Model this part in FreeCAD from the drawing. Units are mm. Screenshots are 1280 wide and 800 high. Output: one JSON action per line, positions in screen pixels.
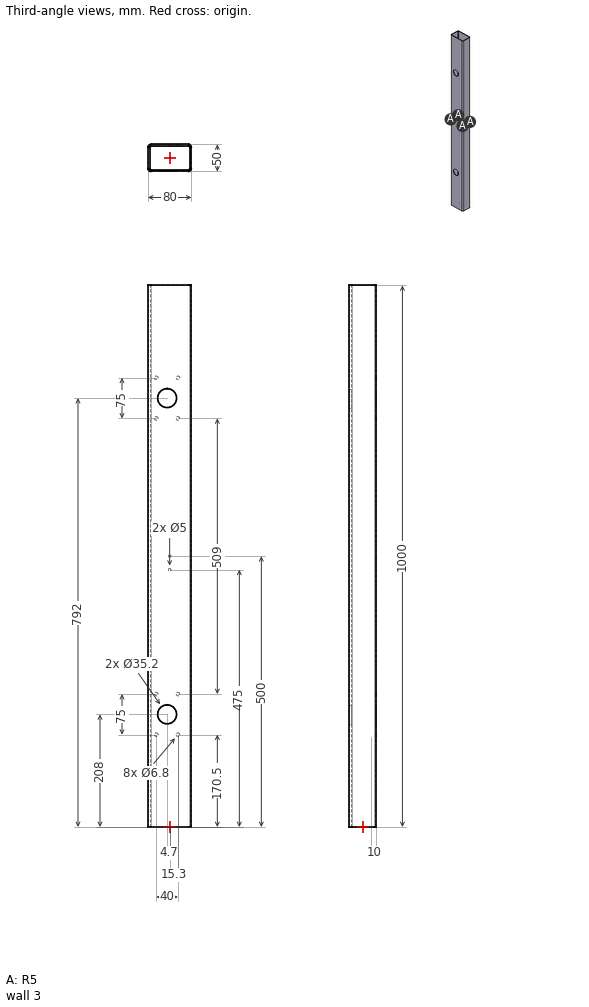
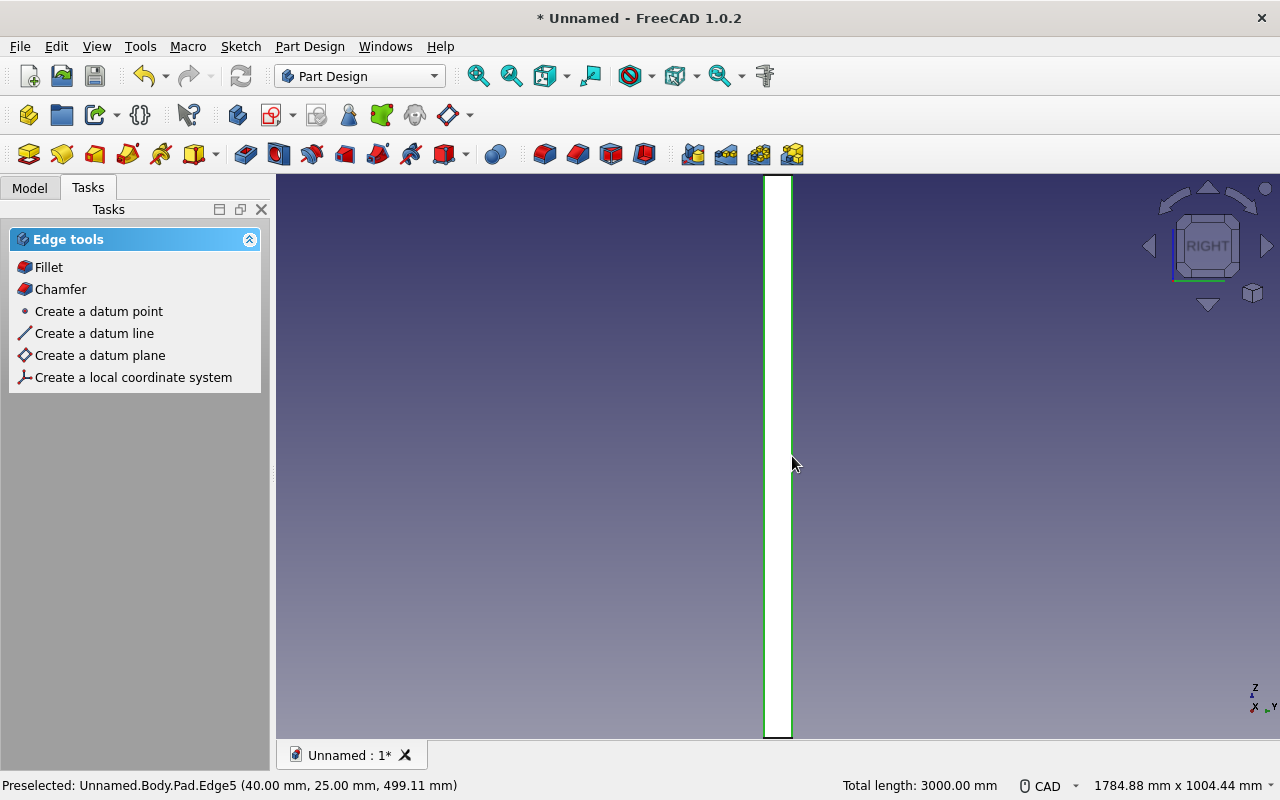
{"action": "key", "text": "5"}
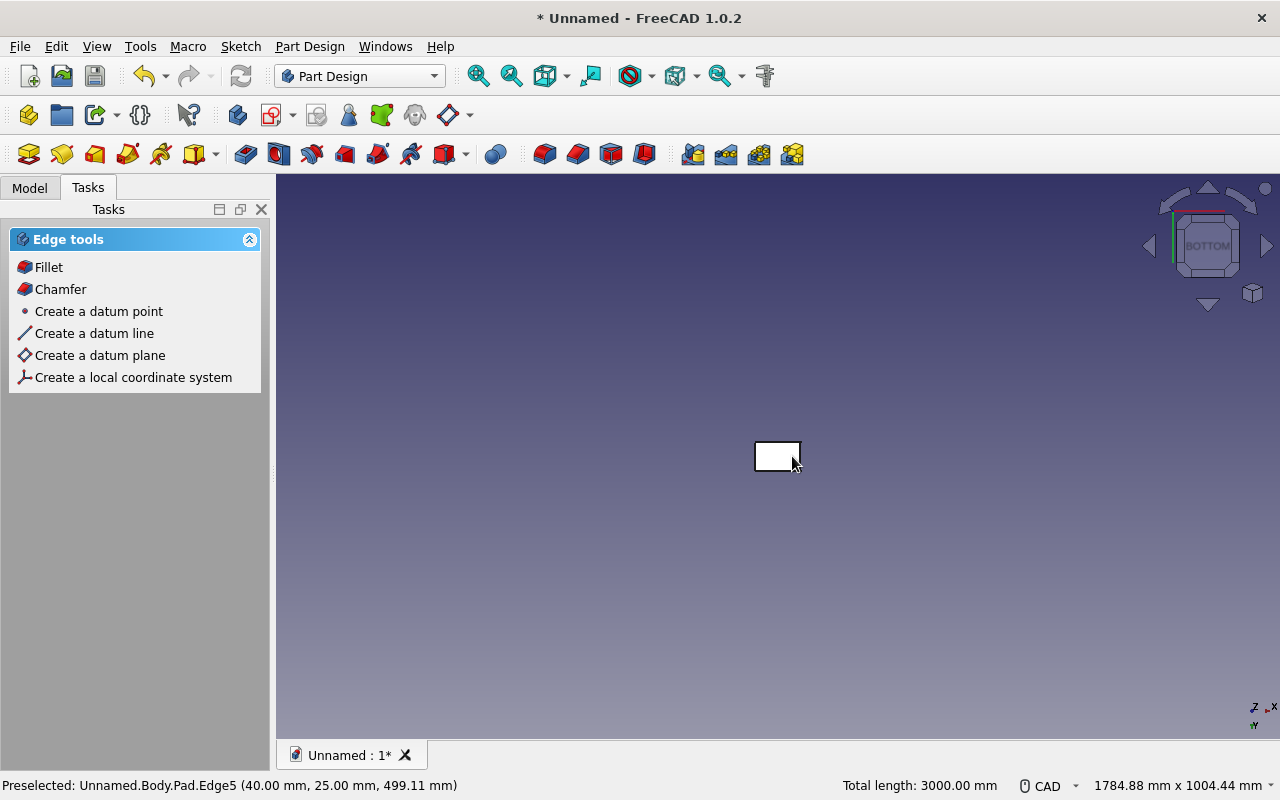
{"action": "left_click", "coordinate": [479, 76]}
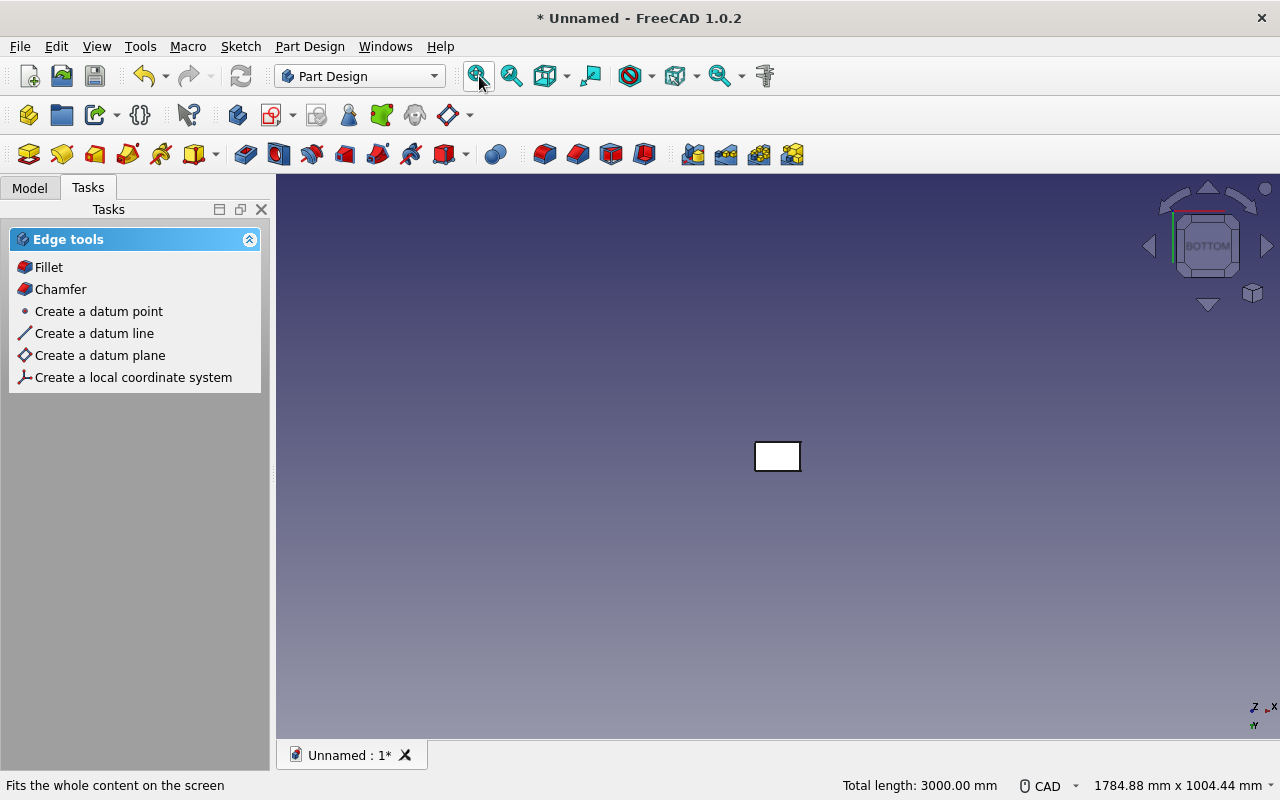
{"action": "key", "text": "4"}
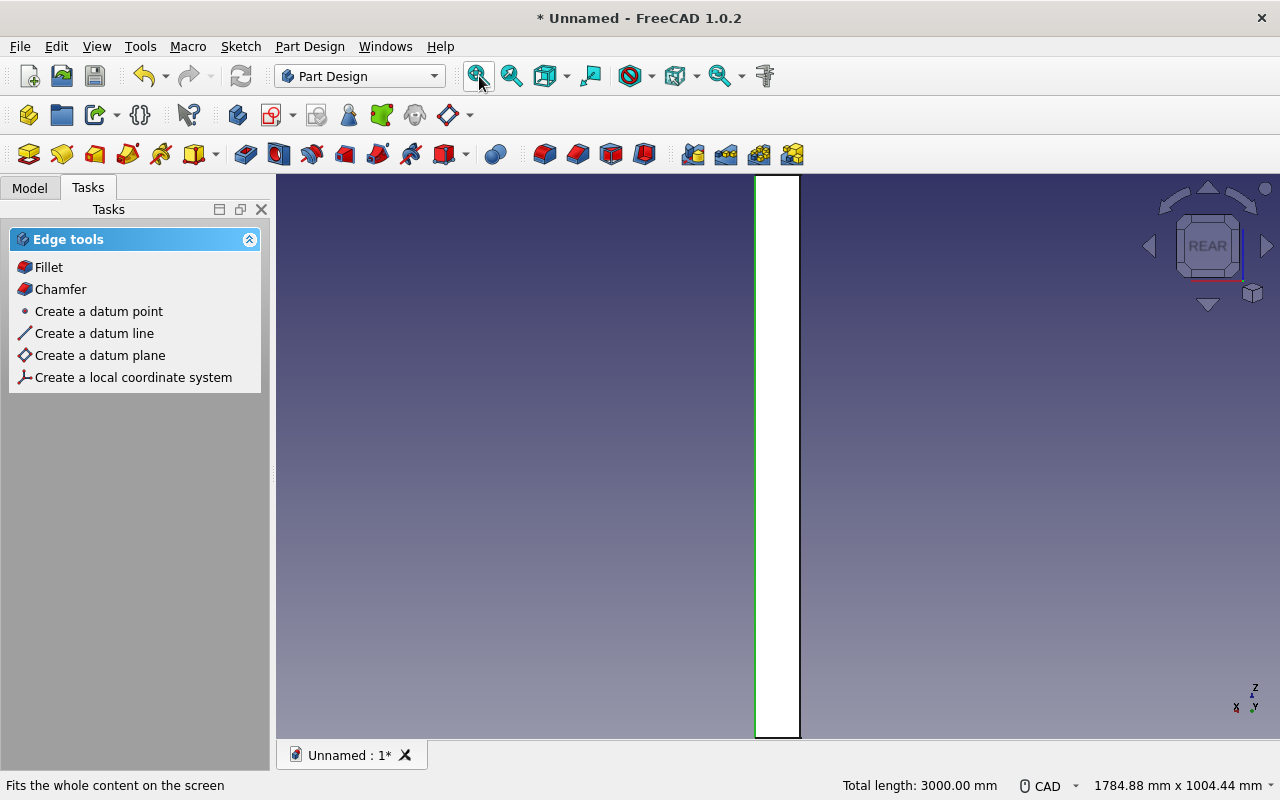
{"action": "left_click", "coordinate": [801, 456], "text": "ctrl"}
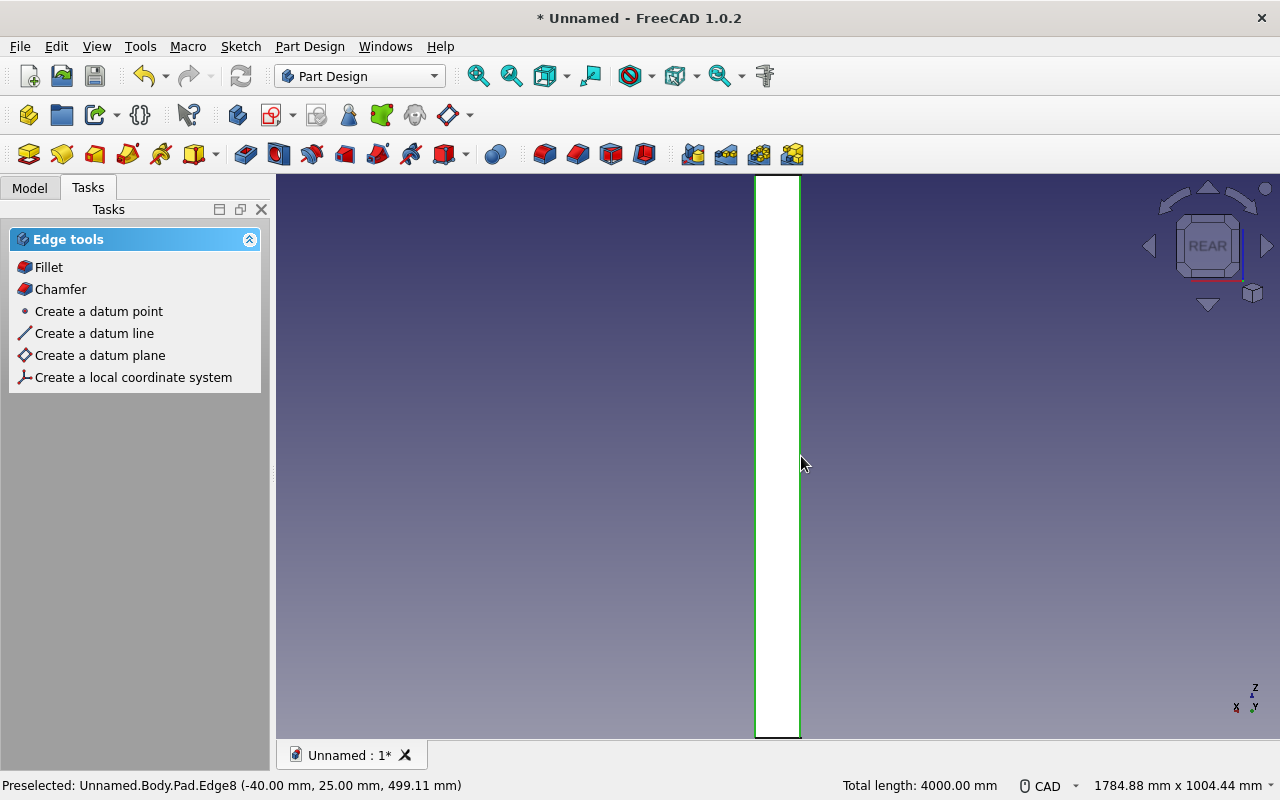
{"action": "left_click", "coordinate": [545, 154]}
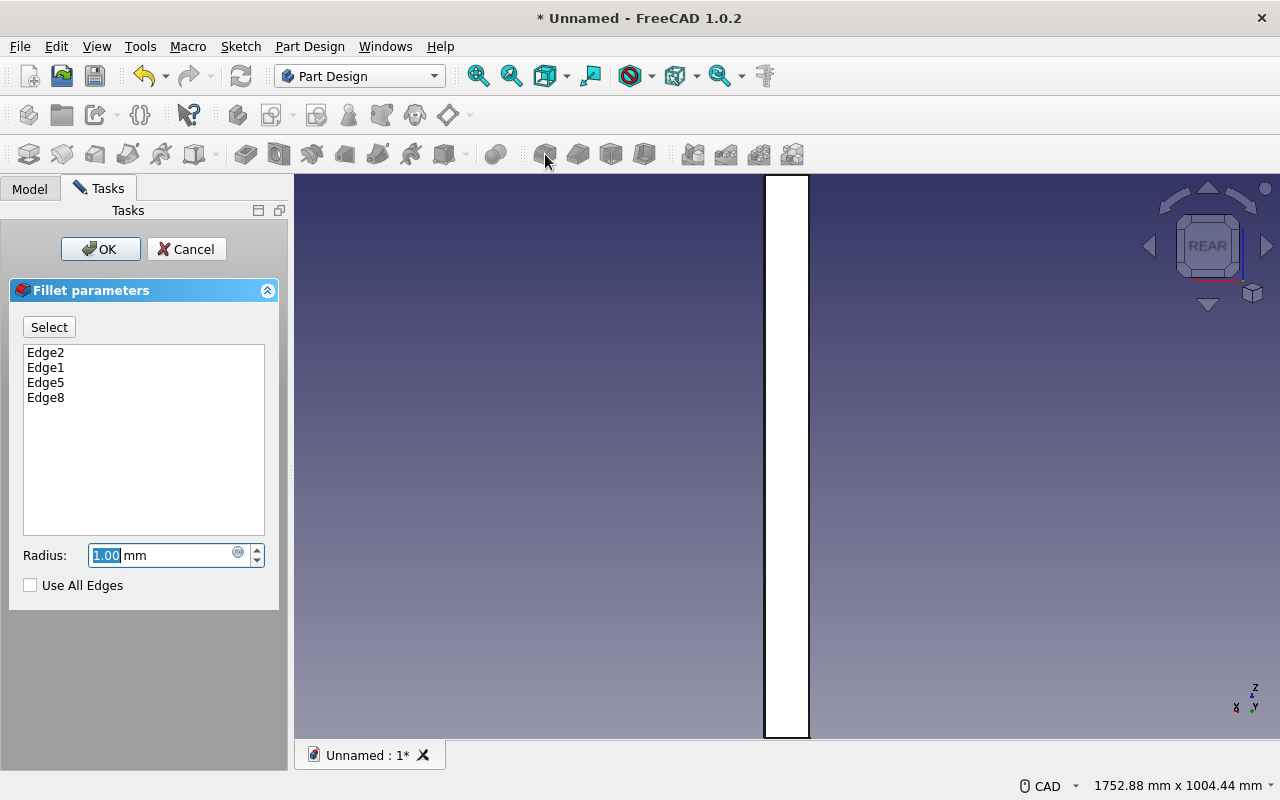
{"action": "type", "text": "5"}
{"action": "key", "text": "Tab"}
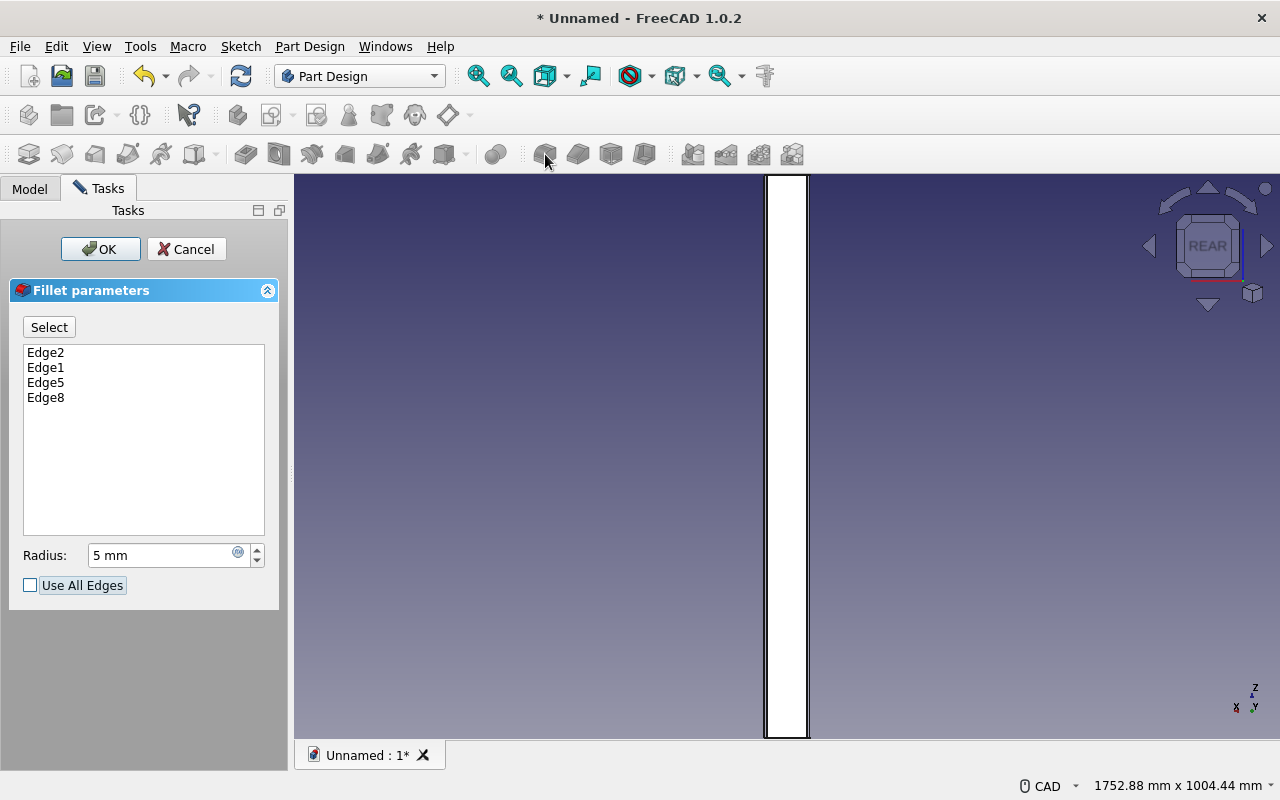
{"action": "left_click", "coordinate": [101, 249]}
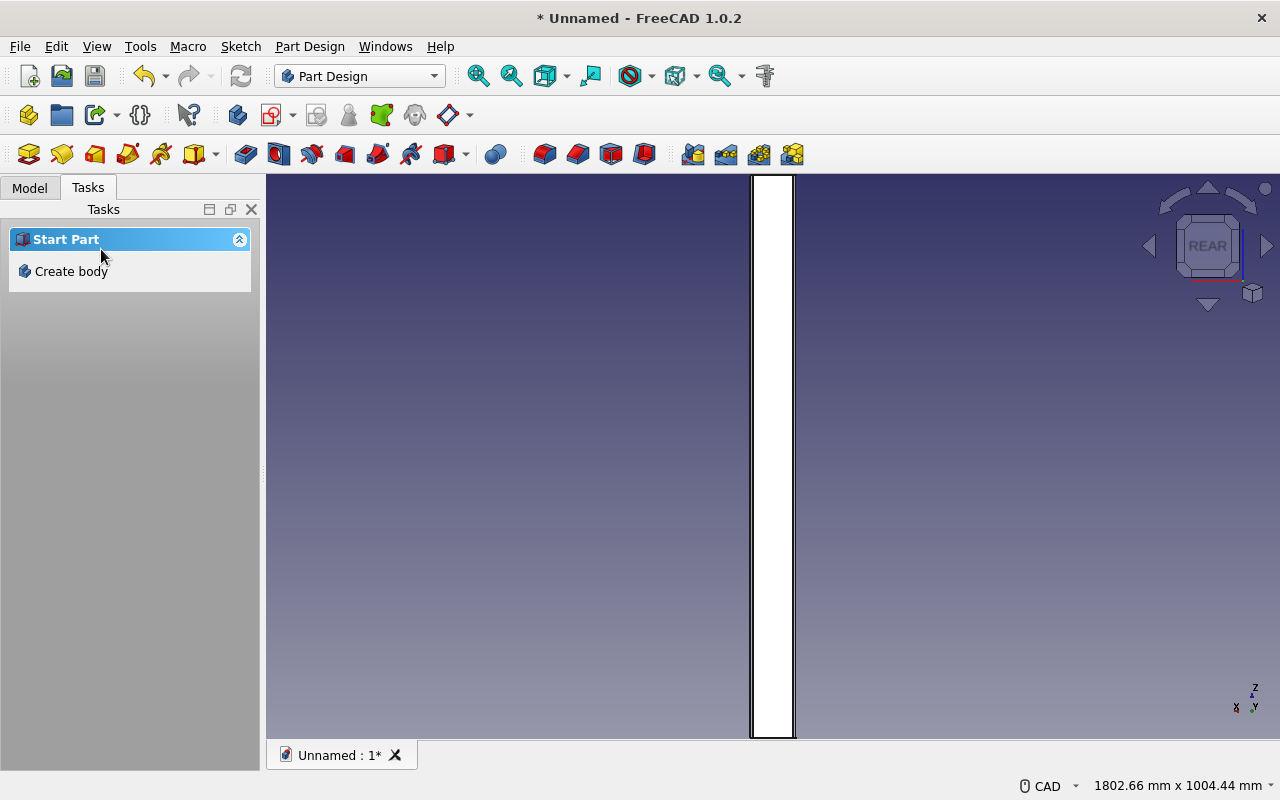
{"action": "key", "text": "0"}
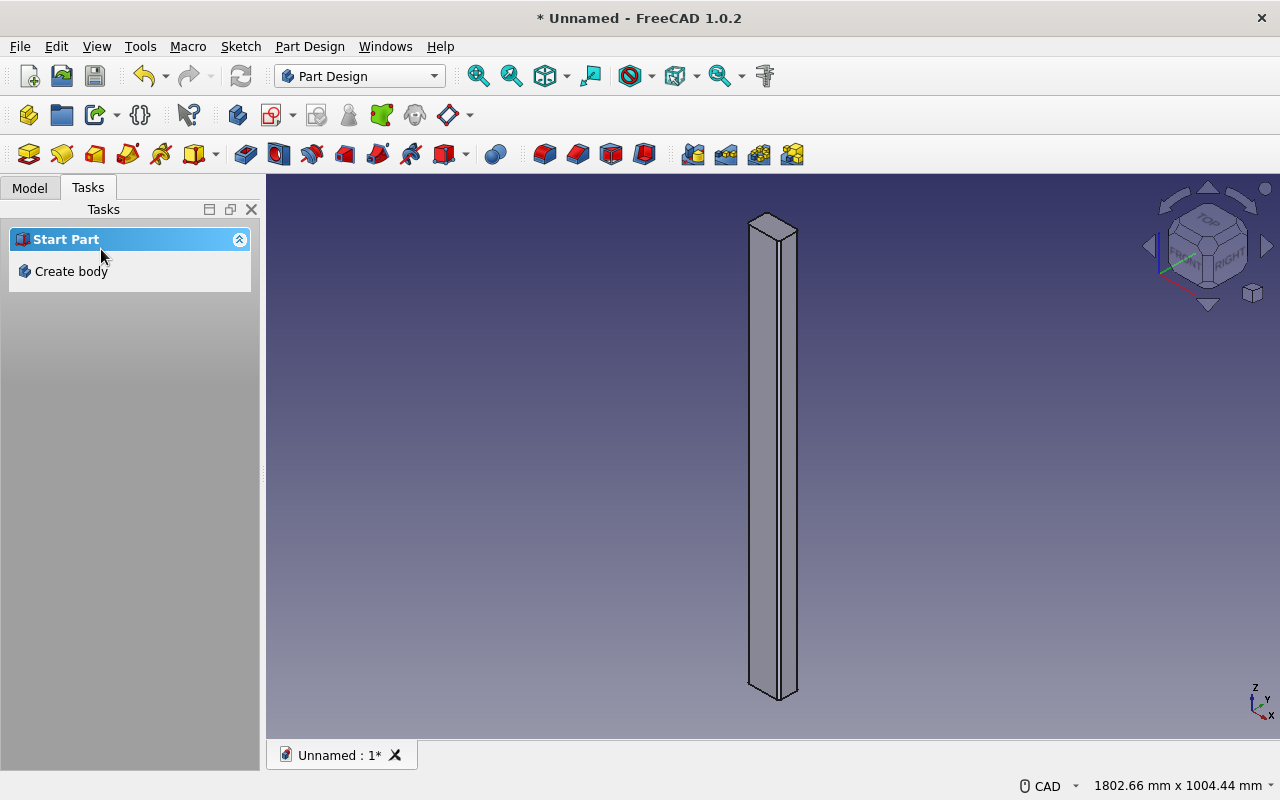
{"action": "left_click", "coordinate": [778, 228]}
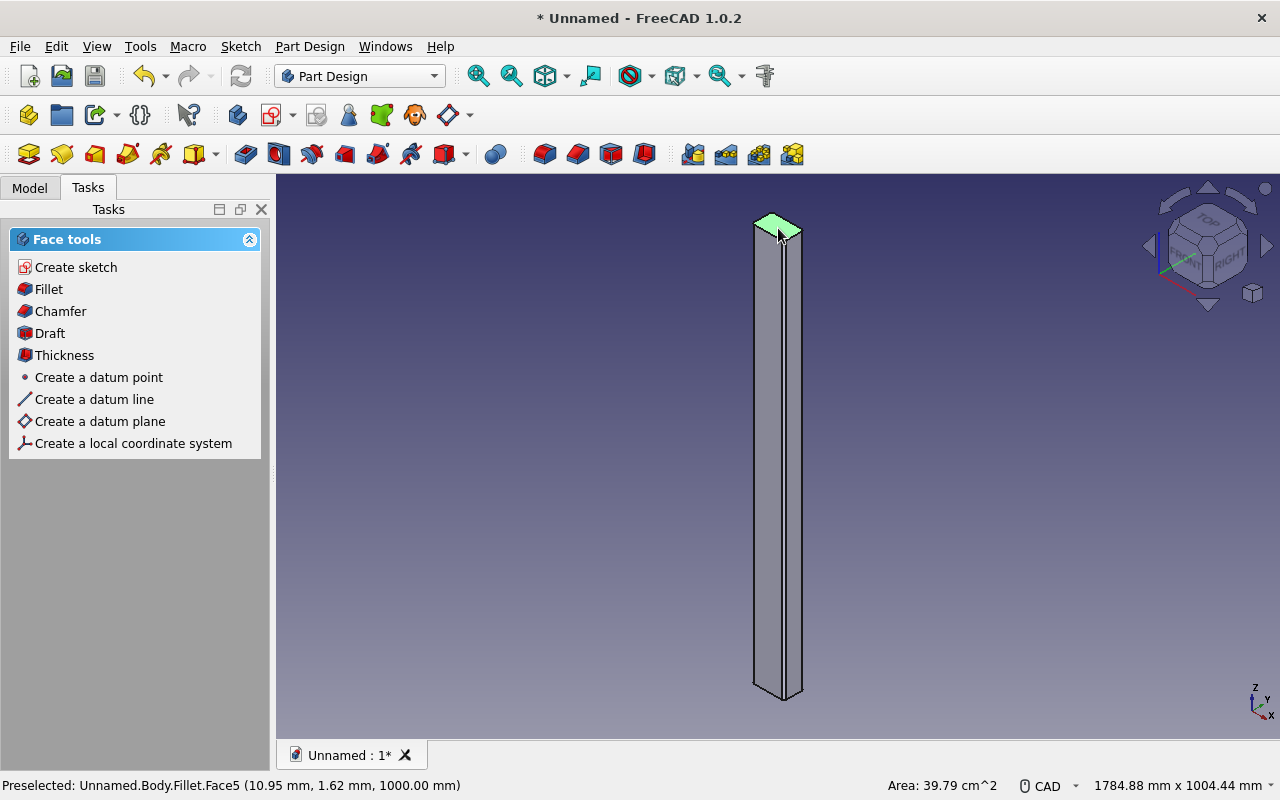
{"action": "key", "text": "2"}